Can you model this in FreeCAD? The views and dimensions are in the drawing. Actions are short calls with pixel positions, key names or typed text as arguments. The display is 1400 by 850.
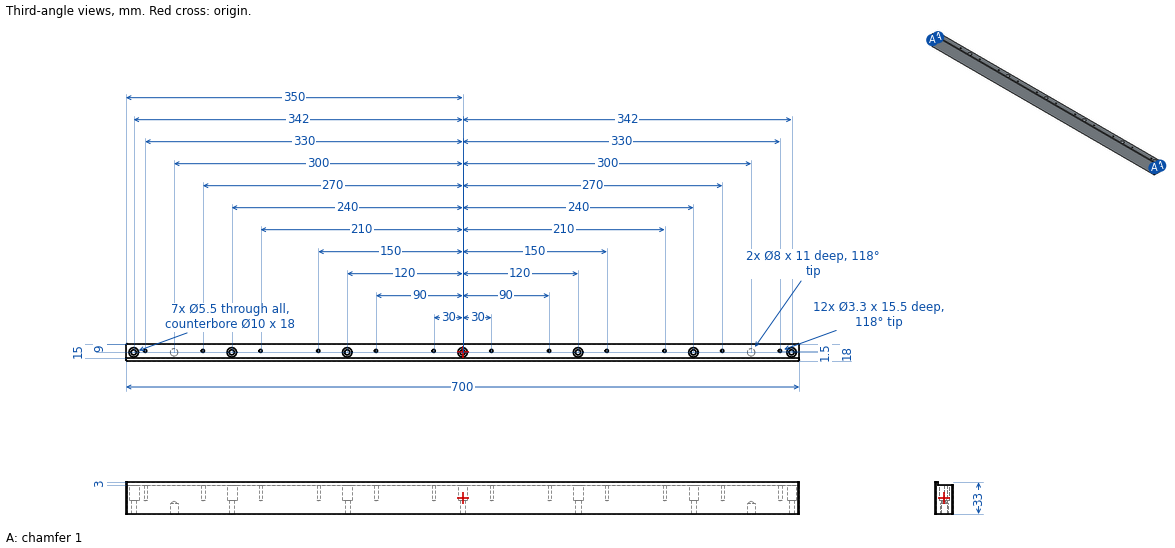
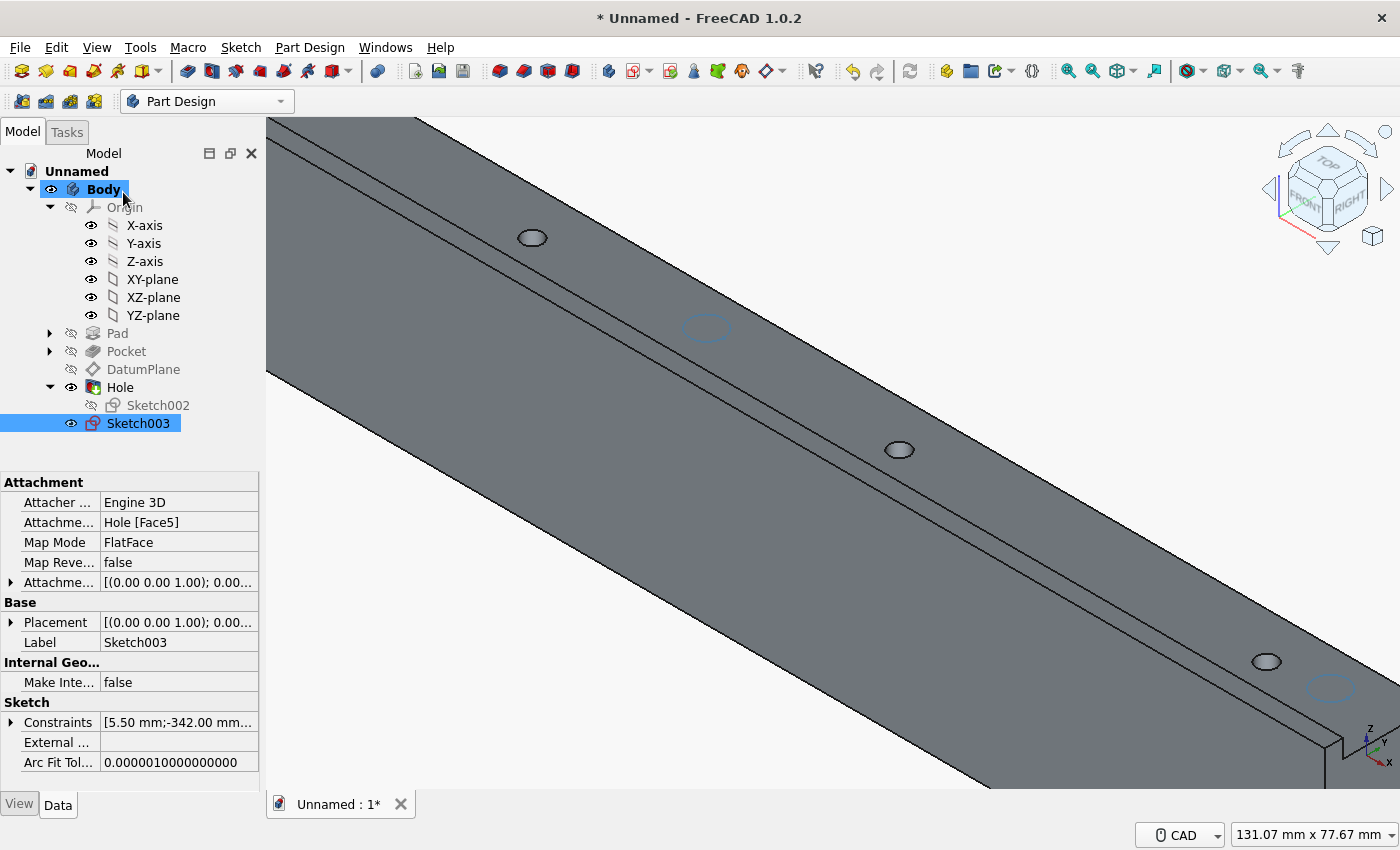
click(212, 72)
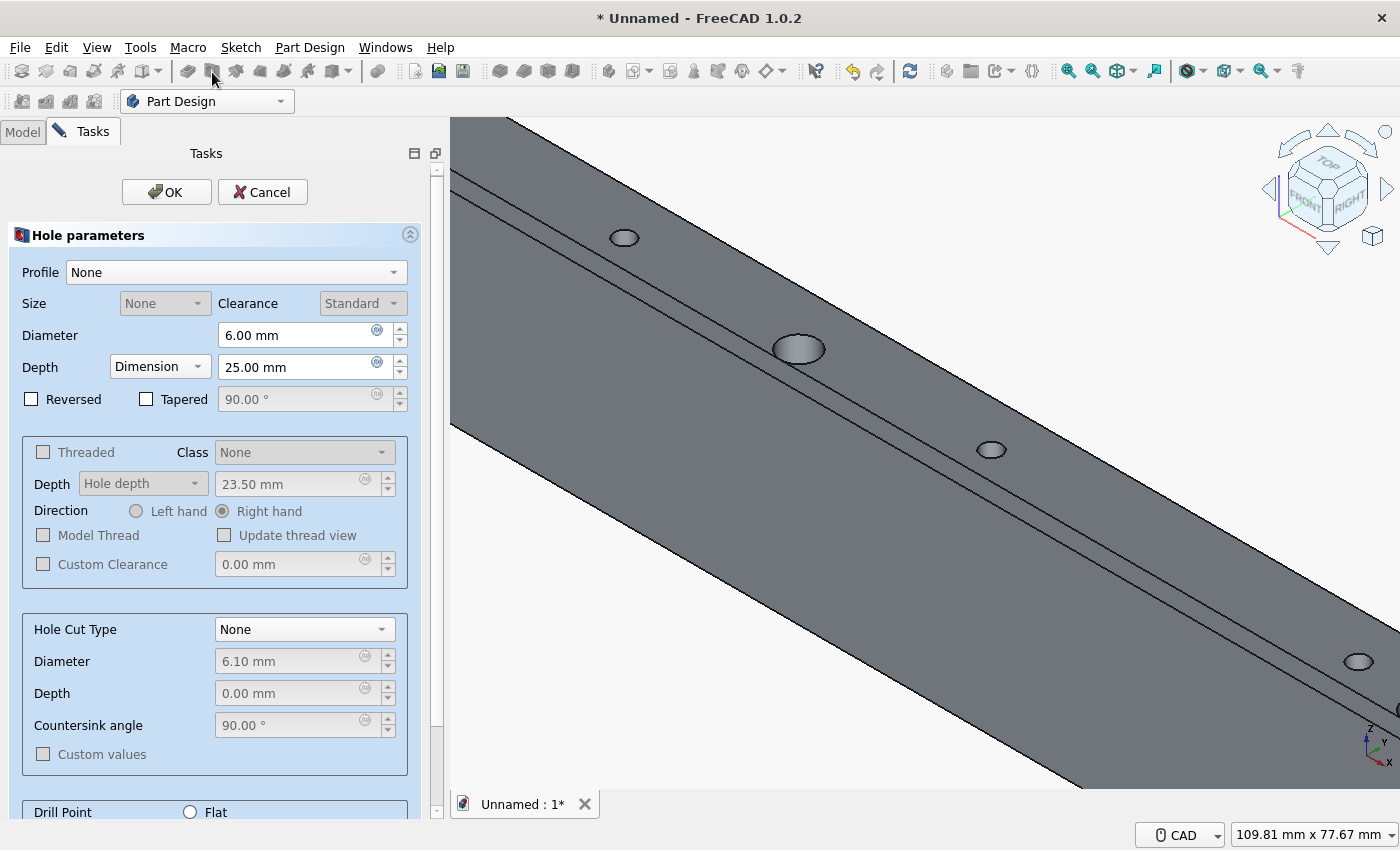
triple_click(305, 335)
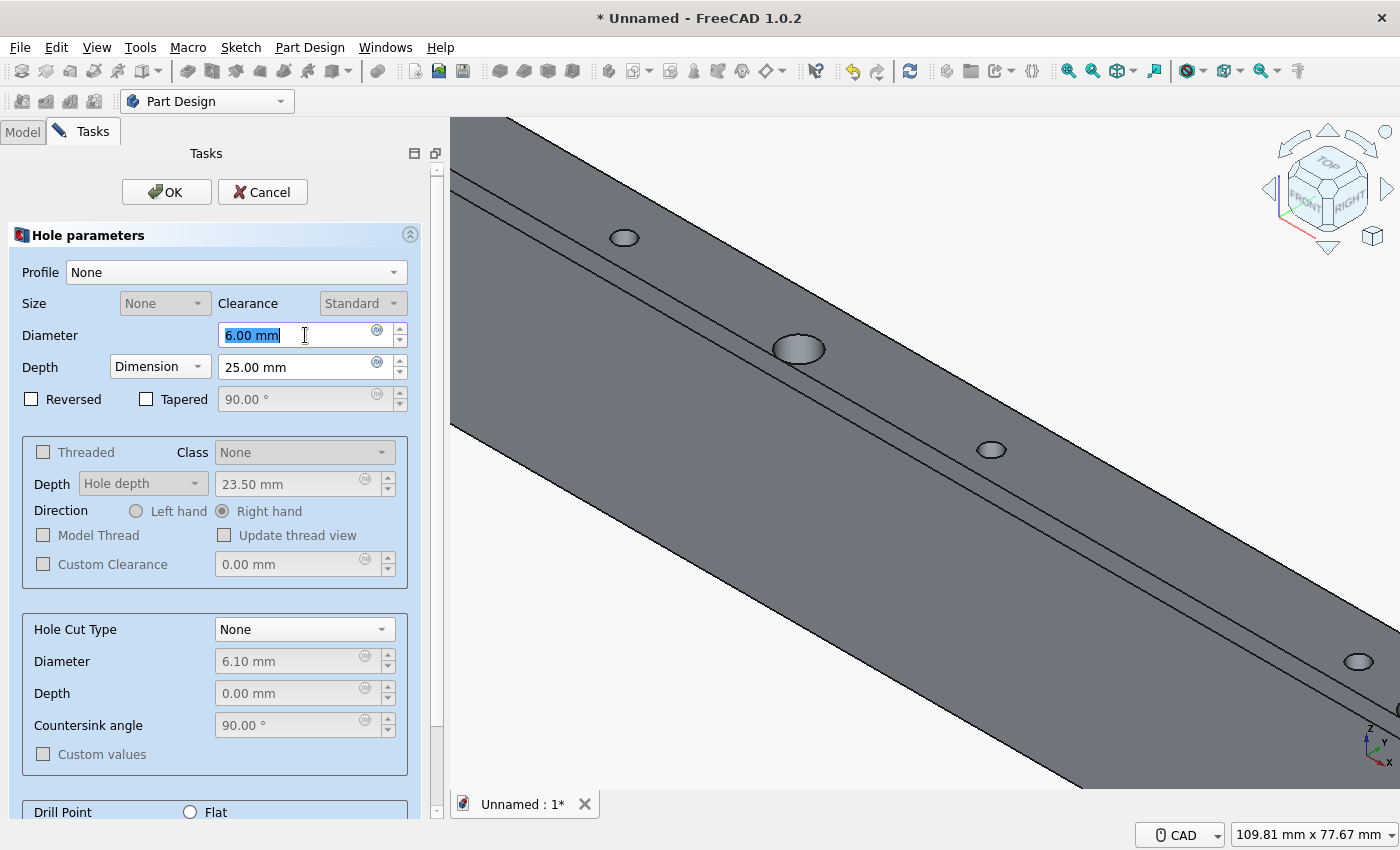
text(5.5)
key(Tab)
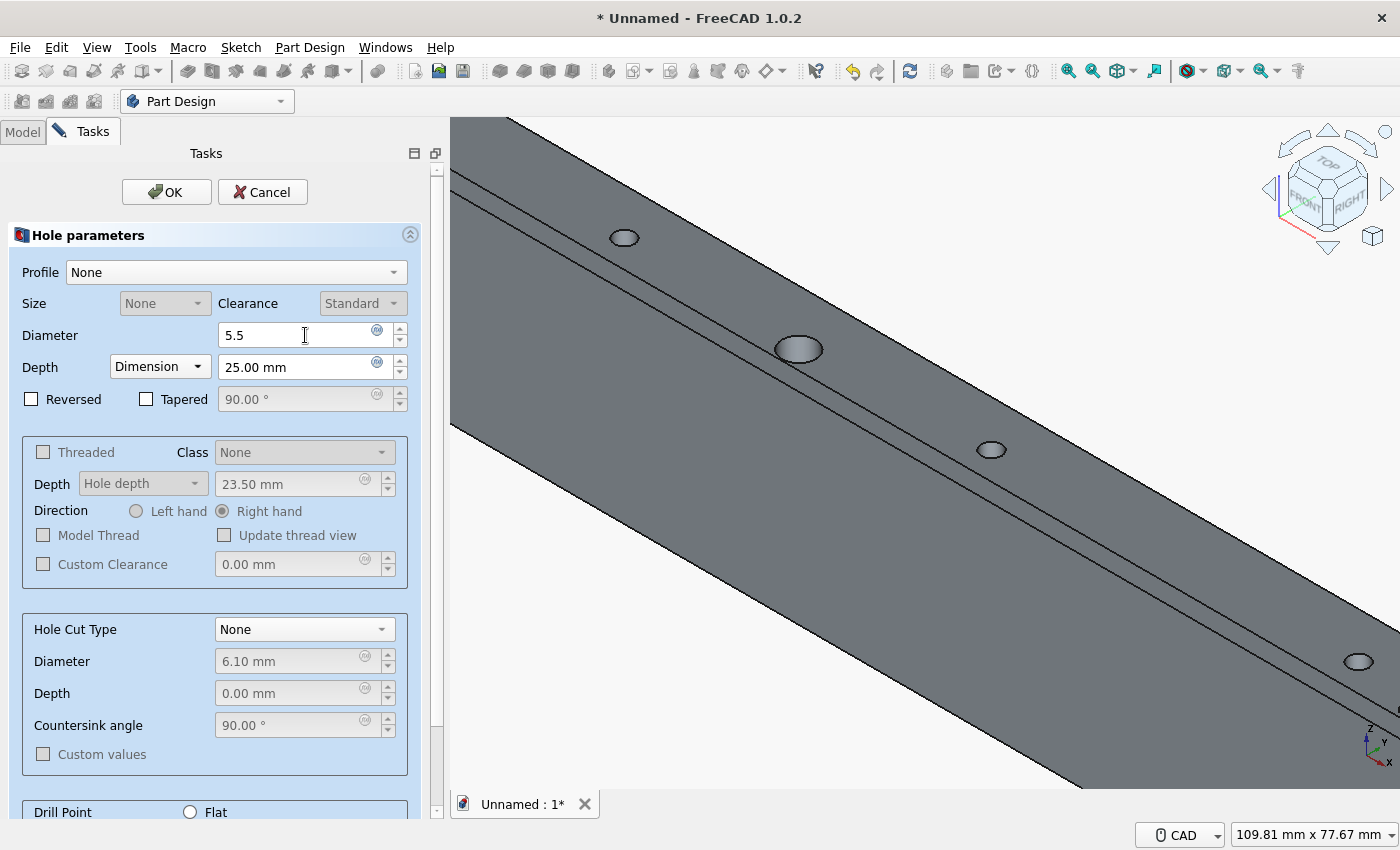
click(161, 366)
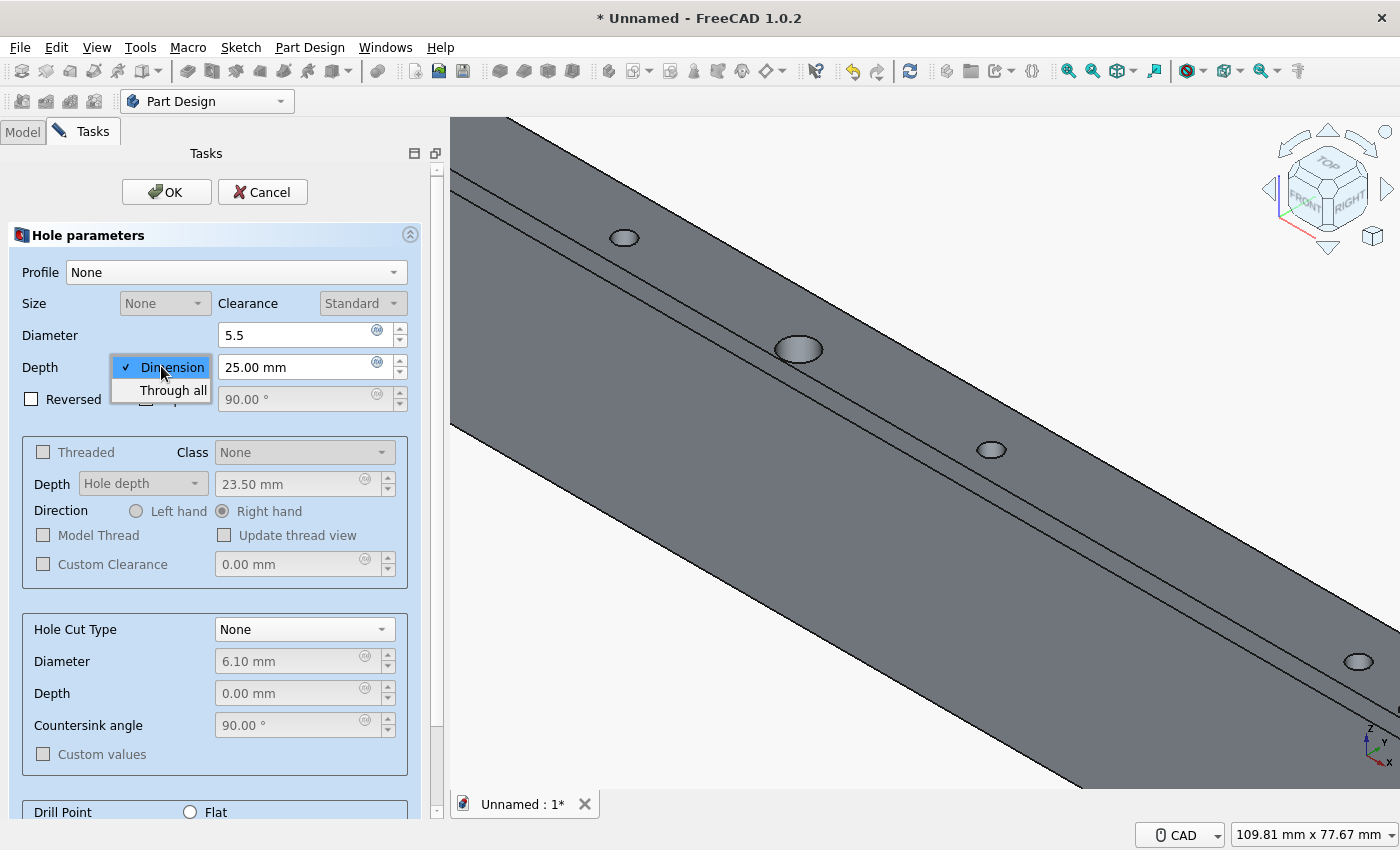
click(160, 390)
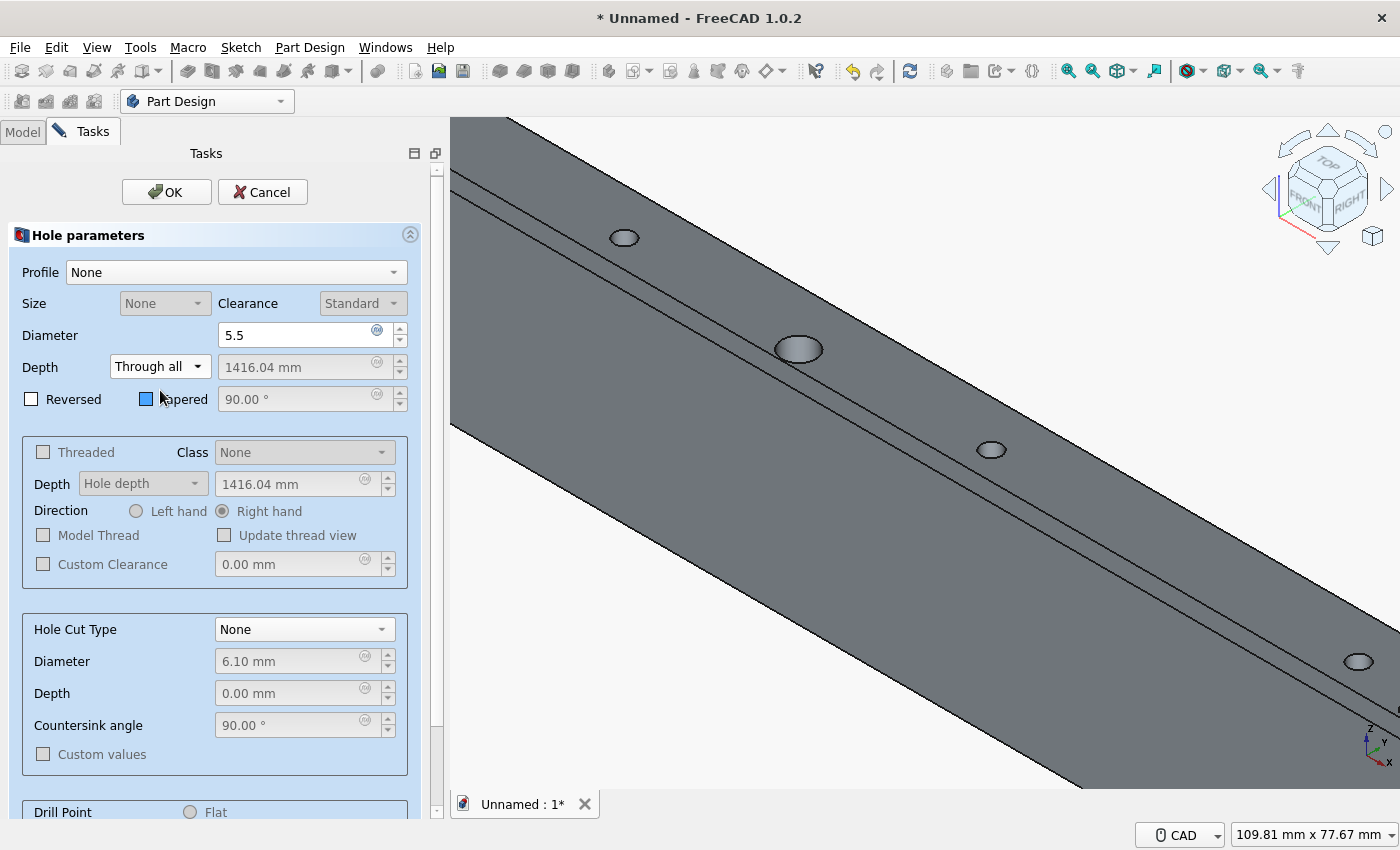
click(306, 630)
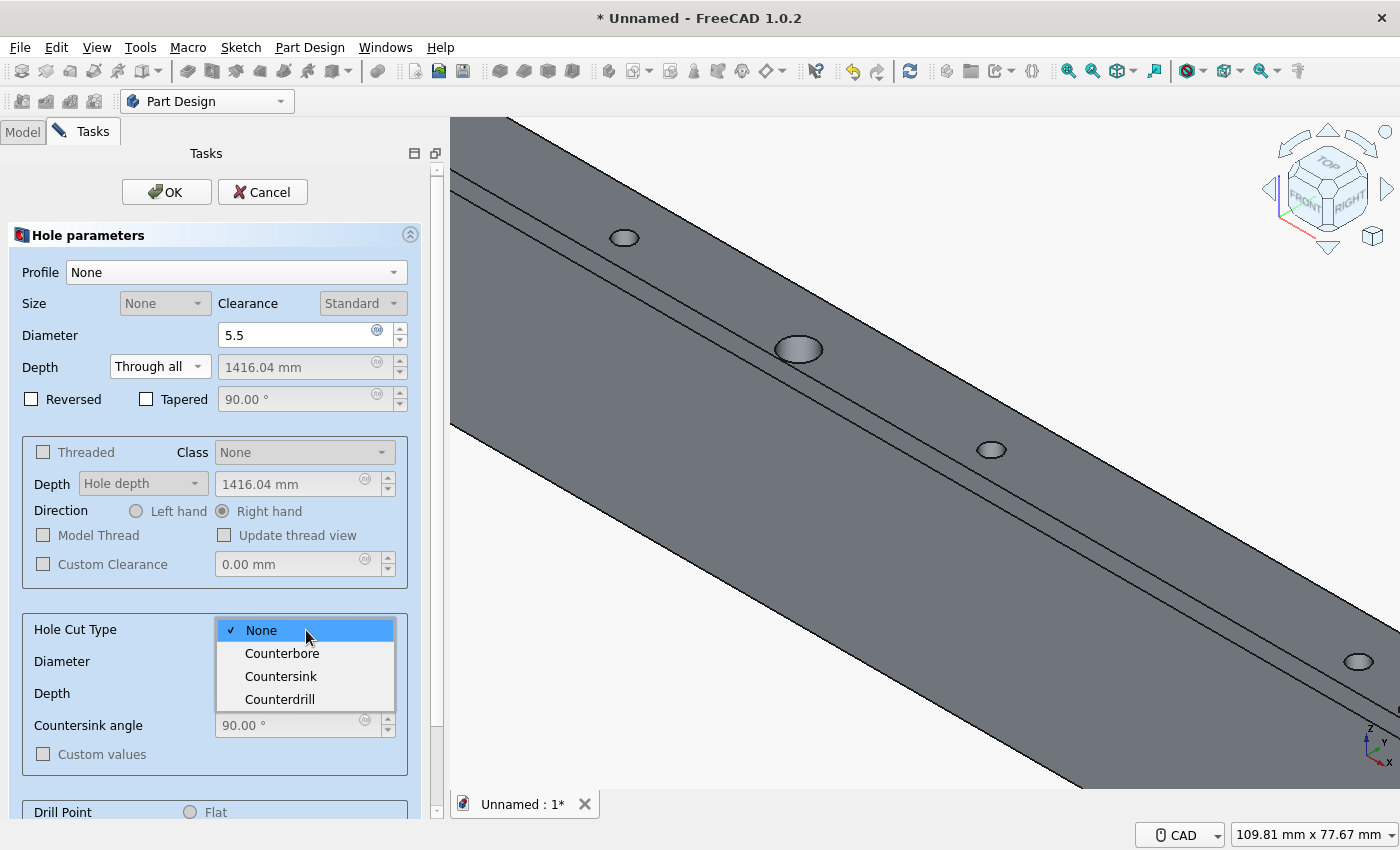
click(304, 654)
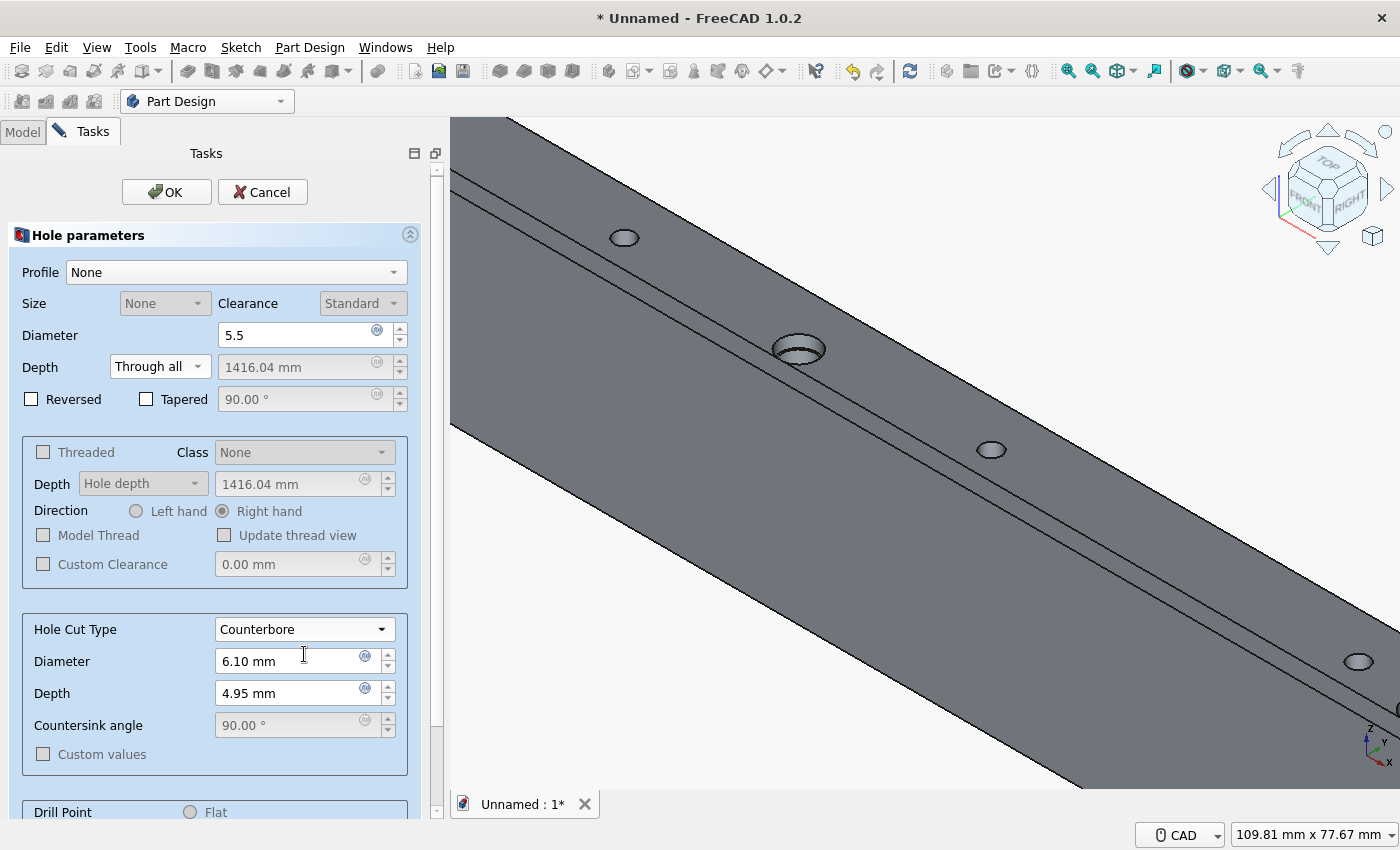
triple_click(298, 661)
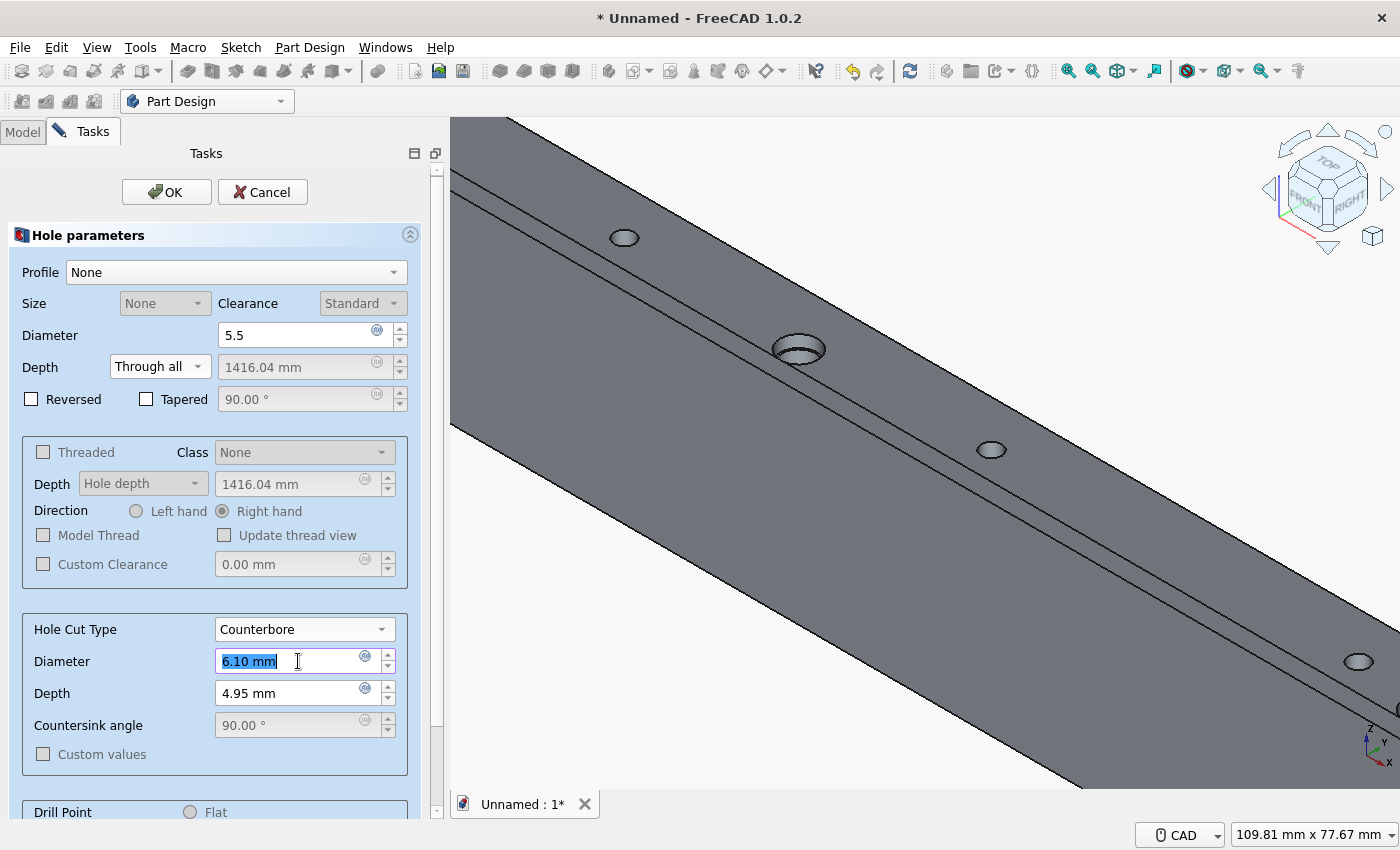
text(10)
key(Tab)